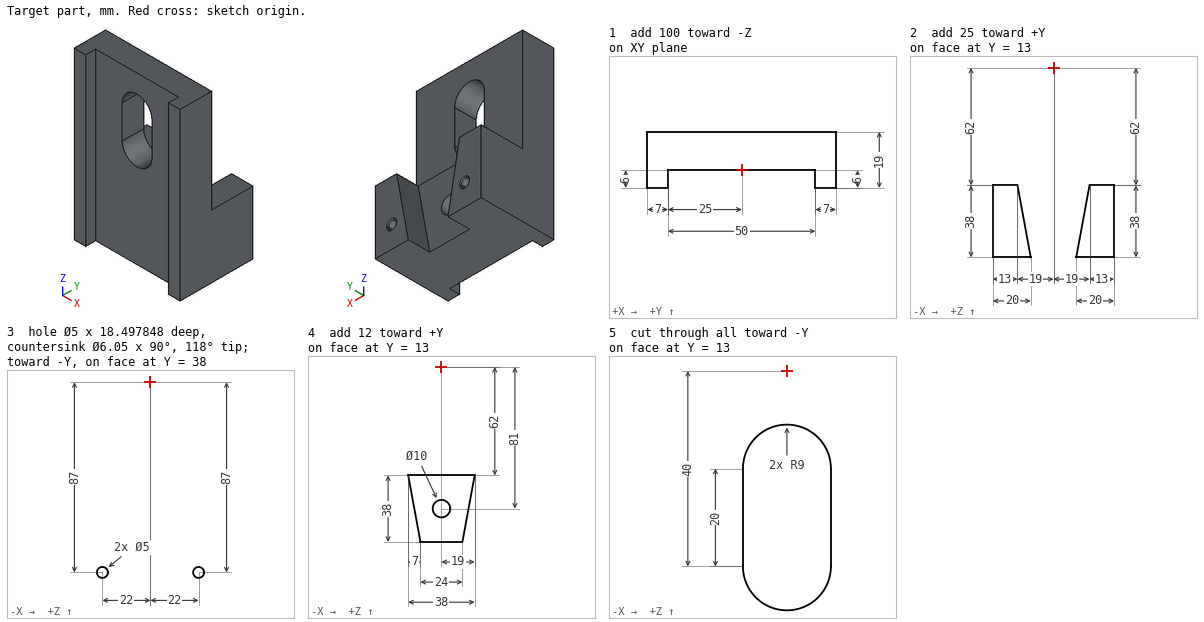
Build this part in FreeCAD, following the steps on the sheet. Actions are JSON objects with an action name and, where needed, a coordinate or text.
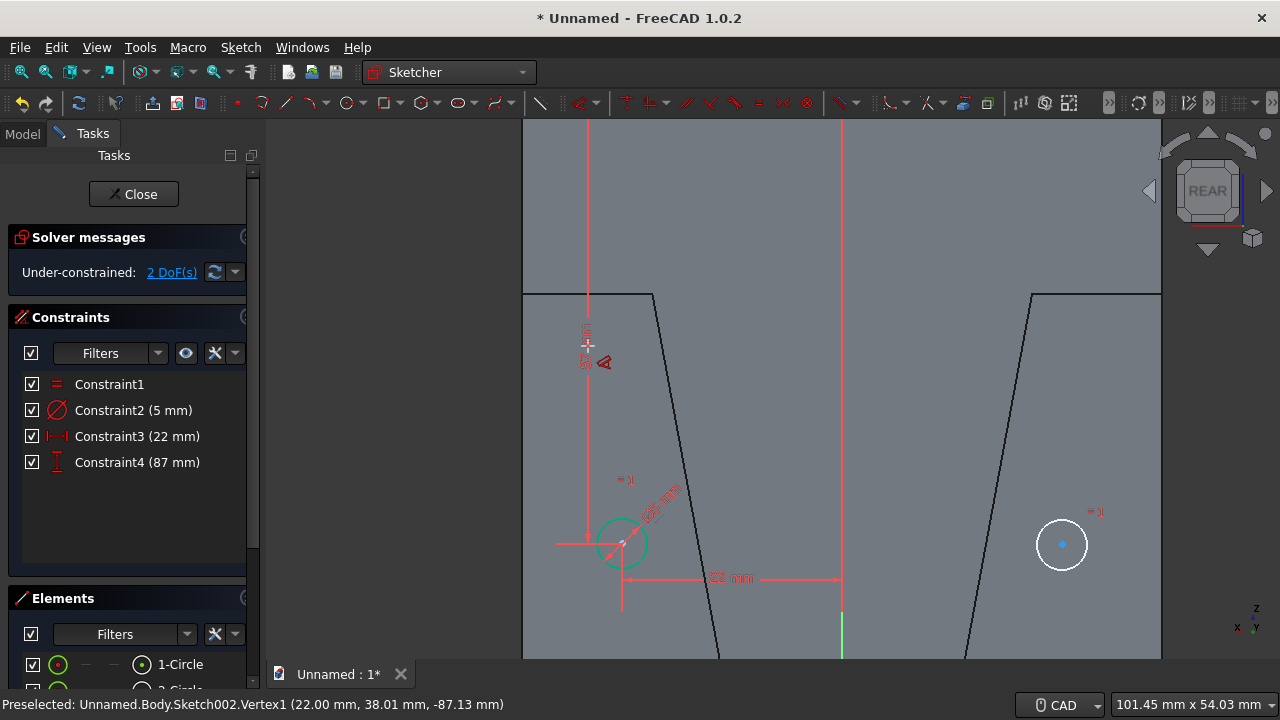
{"action": "left_click", "coordinate": [1062, 545]}
{"action": "left_click", "coordinate": [952, 579]}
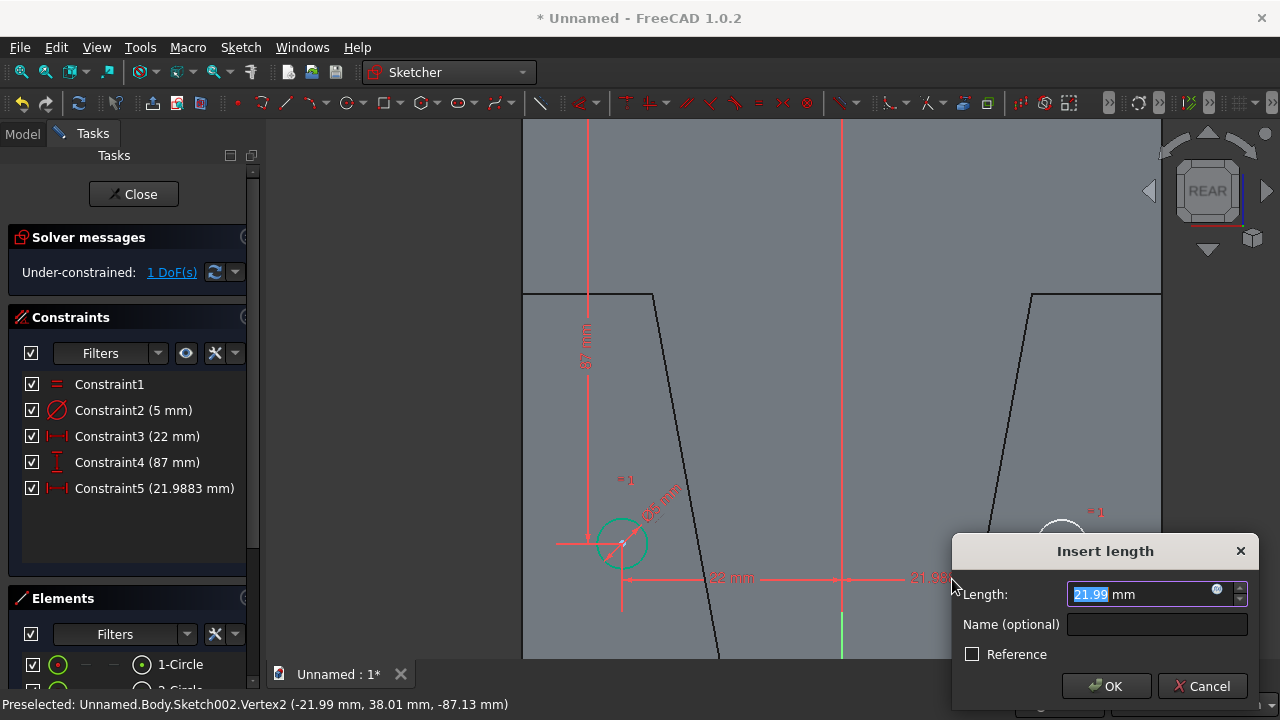
{"action": "type", "text": "22"}
{"action": "key", "text": "Return"}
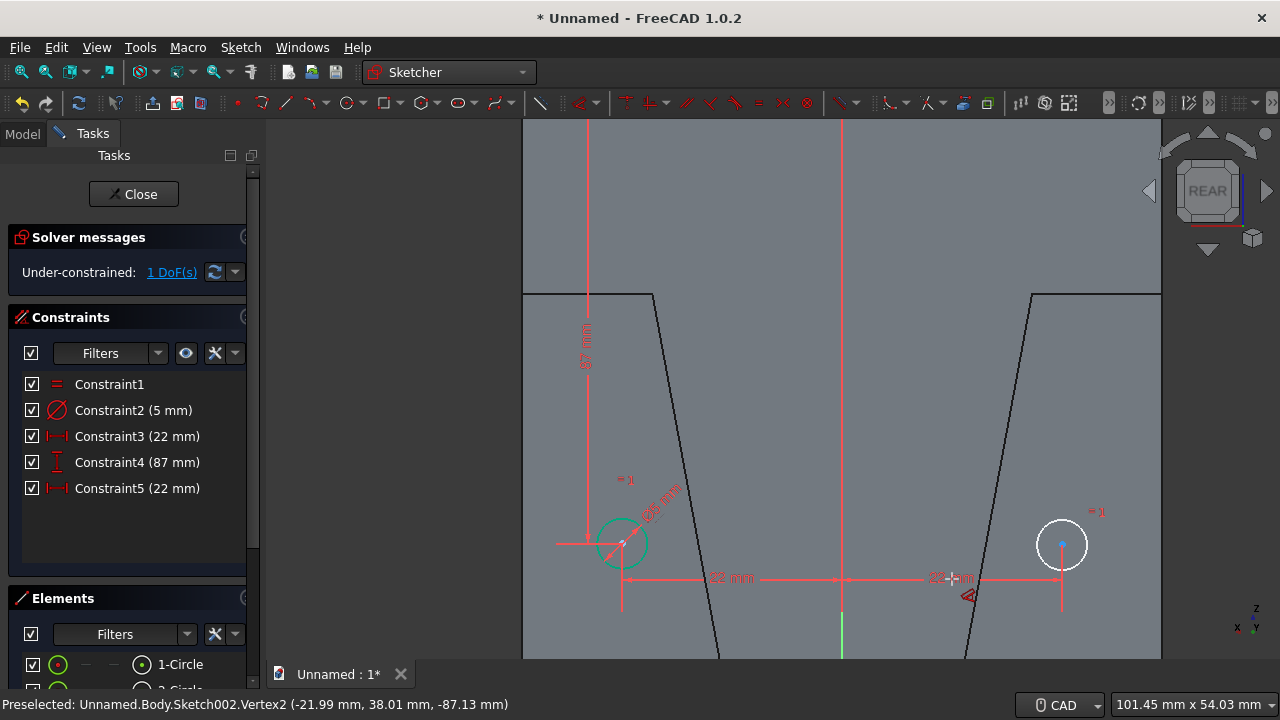
{"action": "left_click", "coordinate": [1062, 545]}
{"action": "left_click", "coordinate": [1096, 346]}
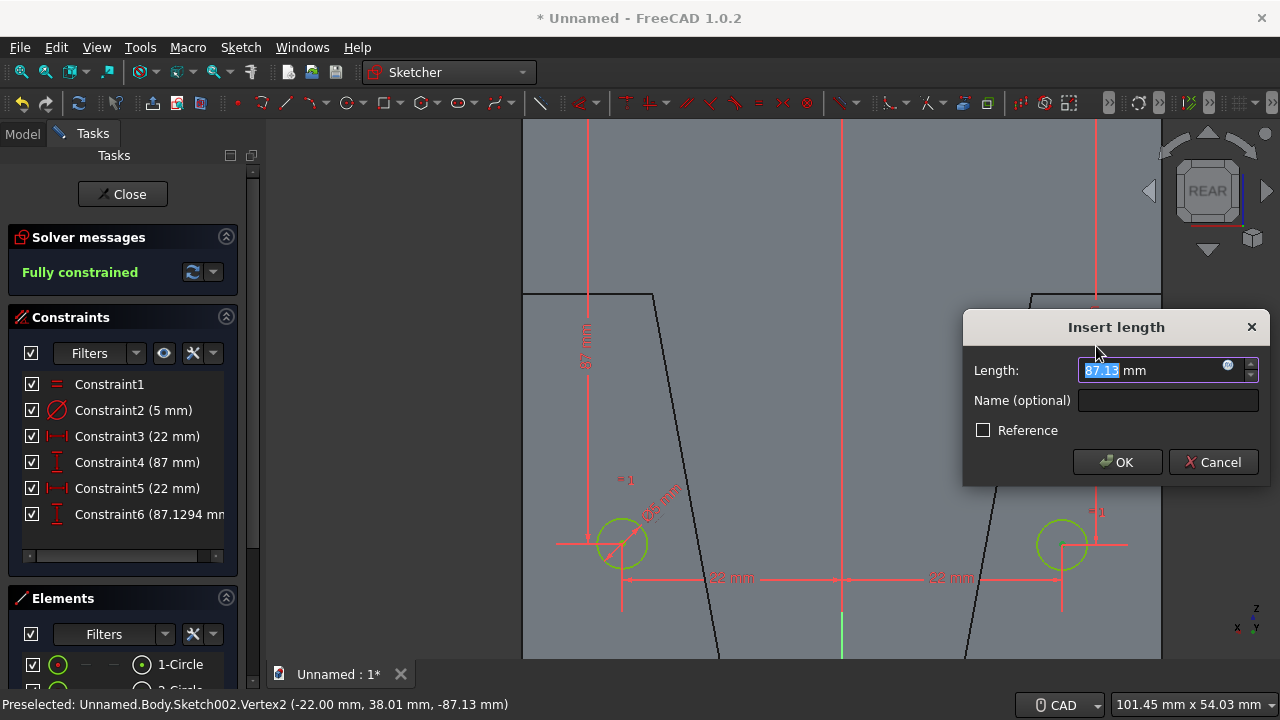
{"action": "type", "text": "87"}
{"action": "key", "text": "Return"}
{"action": "key", "text": "Escape"}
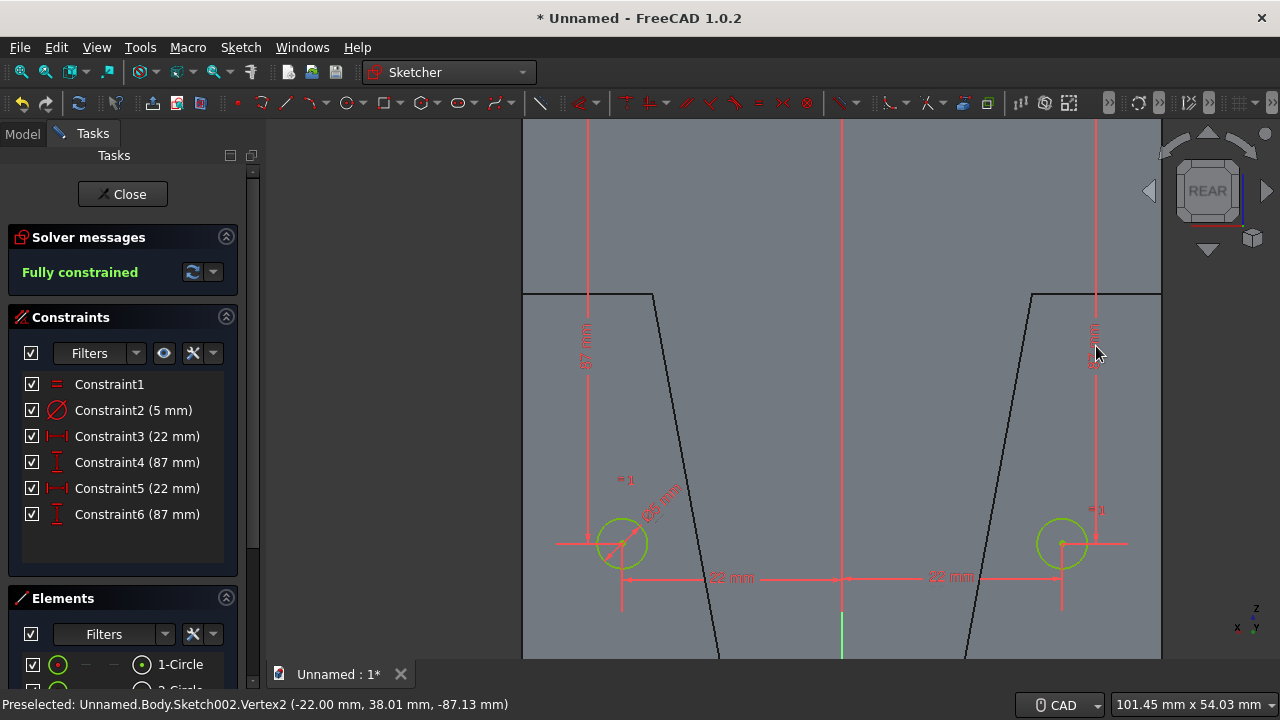
{"action": "left_click", "coordinate": [123, 194]}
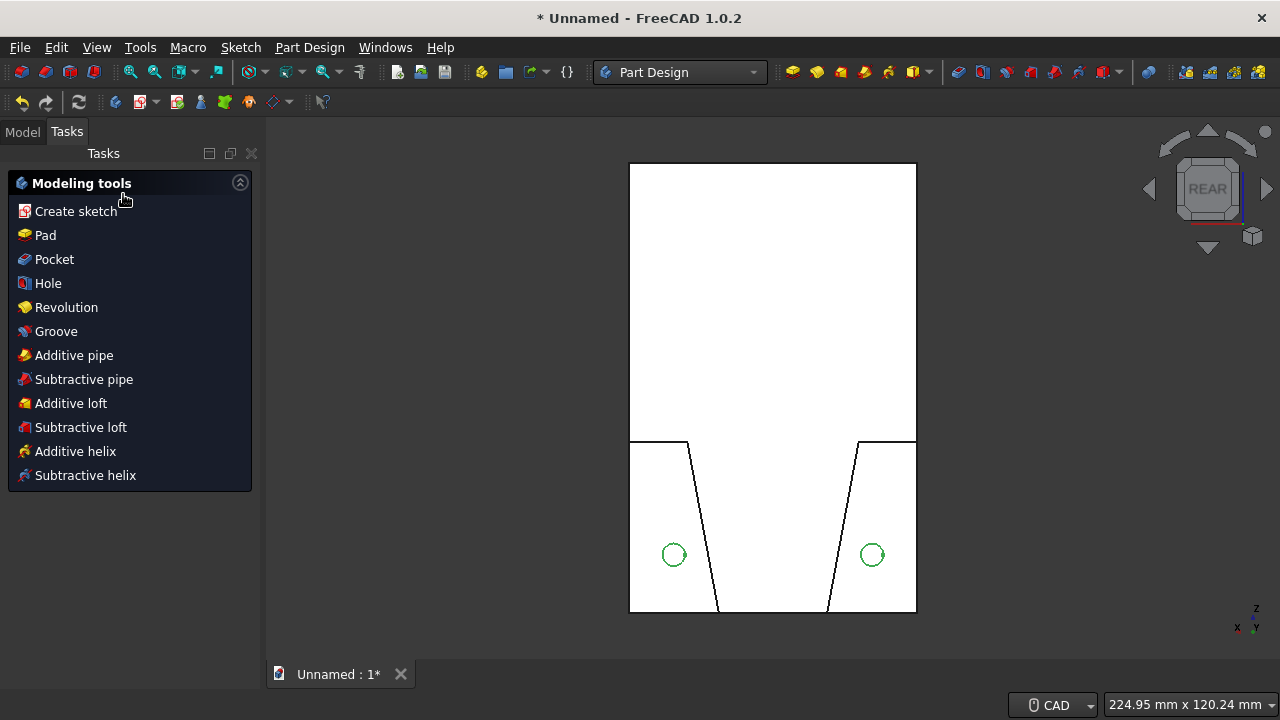
{"action": "left_click", "coordinate": [984, 72]}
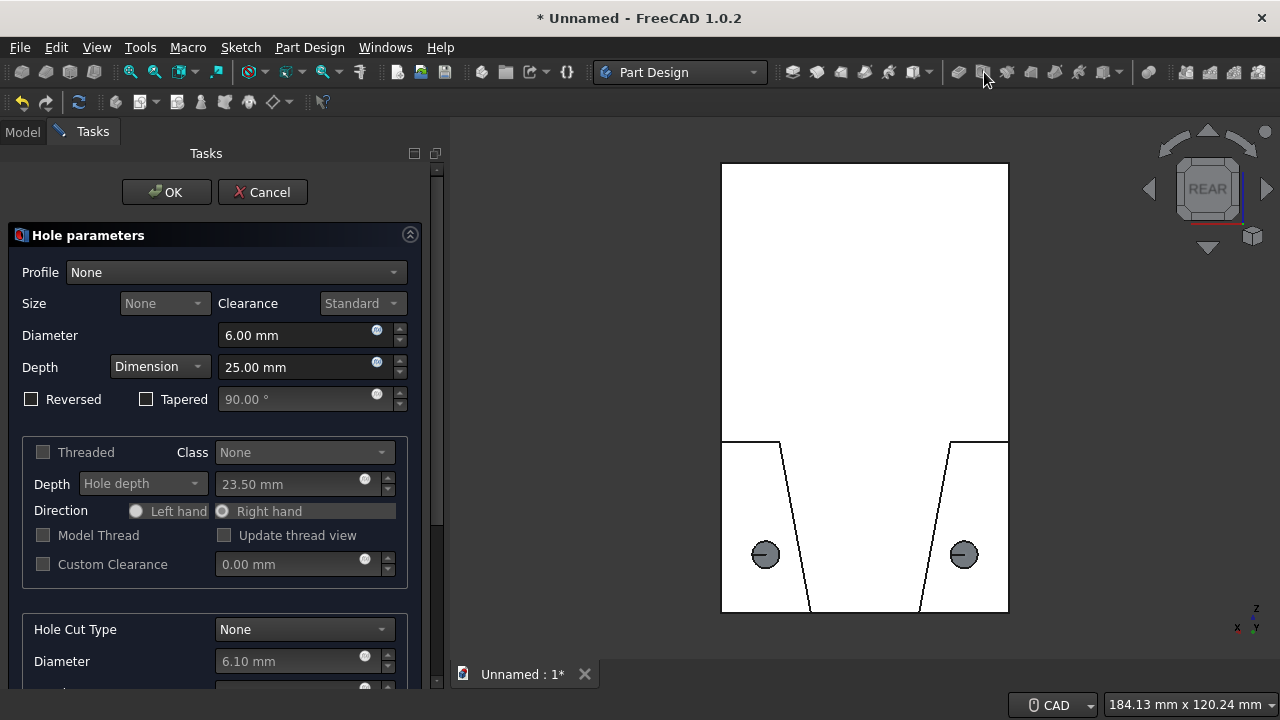
{"action": "triple_click", "coordinate": [305, 335]}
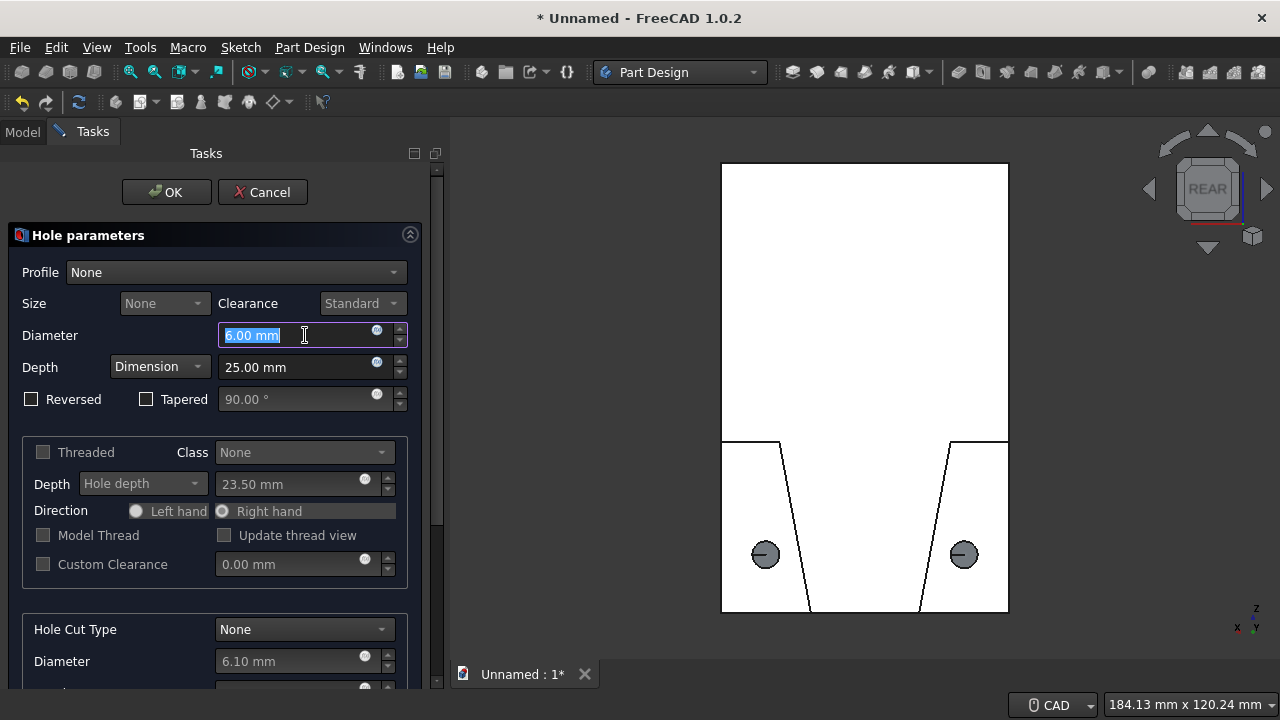
{"action": "type", "text": "5"}
{"action": "key", "text": "Tab"}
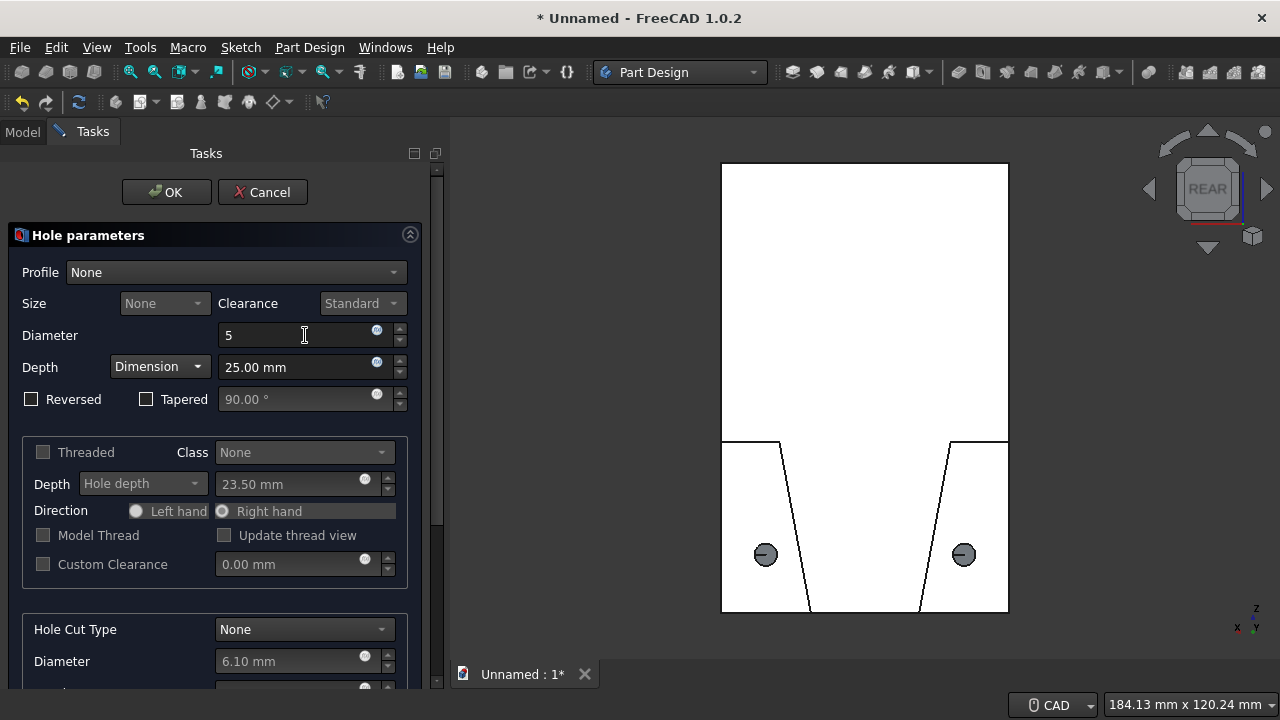
{"action": "triple_click", "coordinate": [305, 367]}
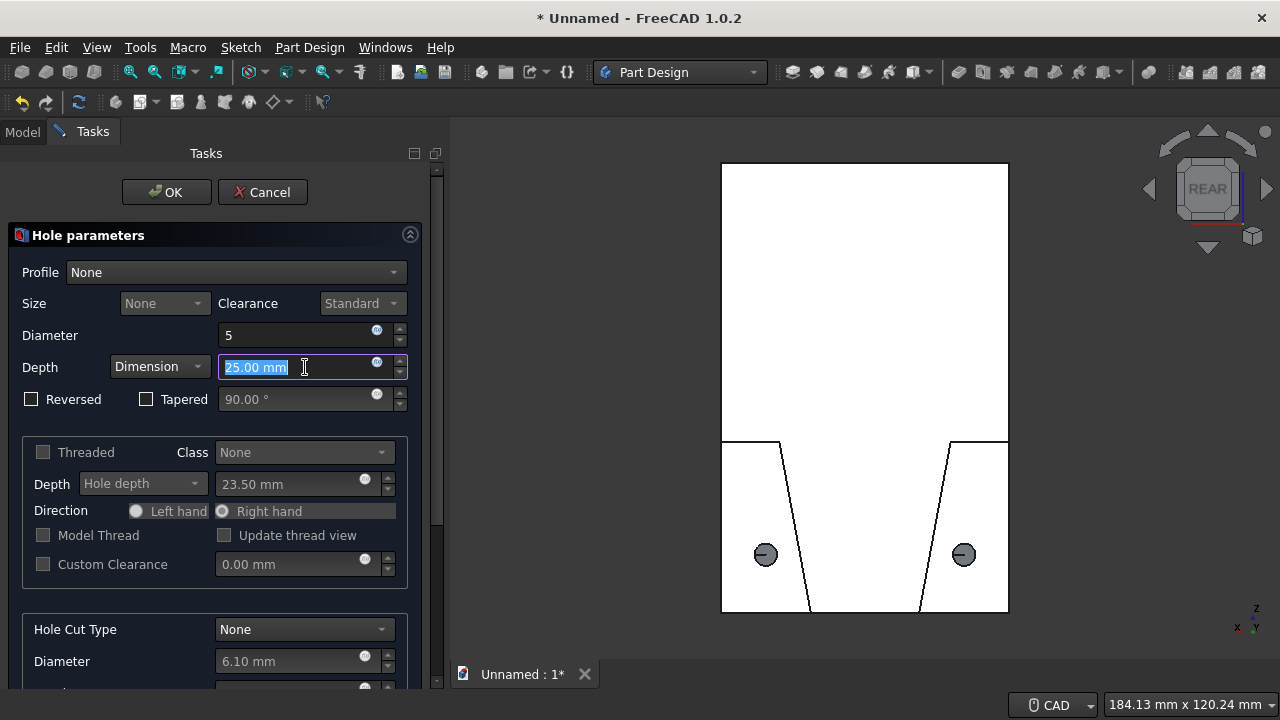
{"action": "type", "text": "18.497848"}
{"action": "key", "text": "Tab"}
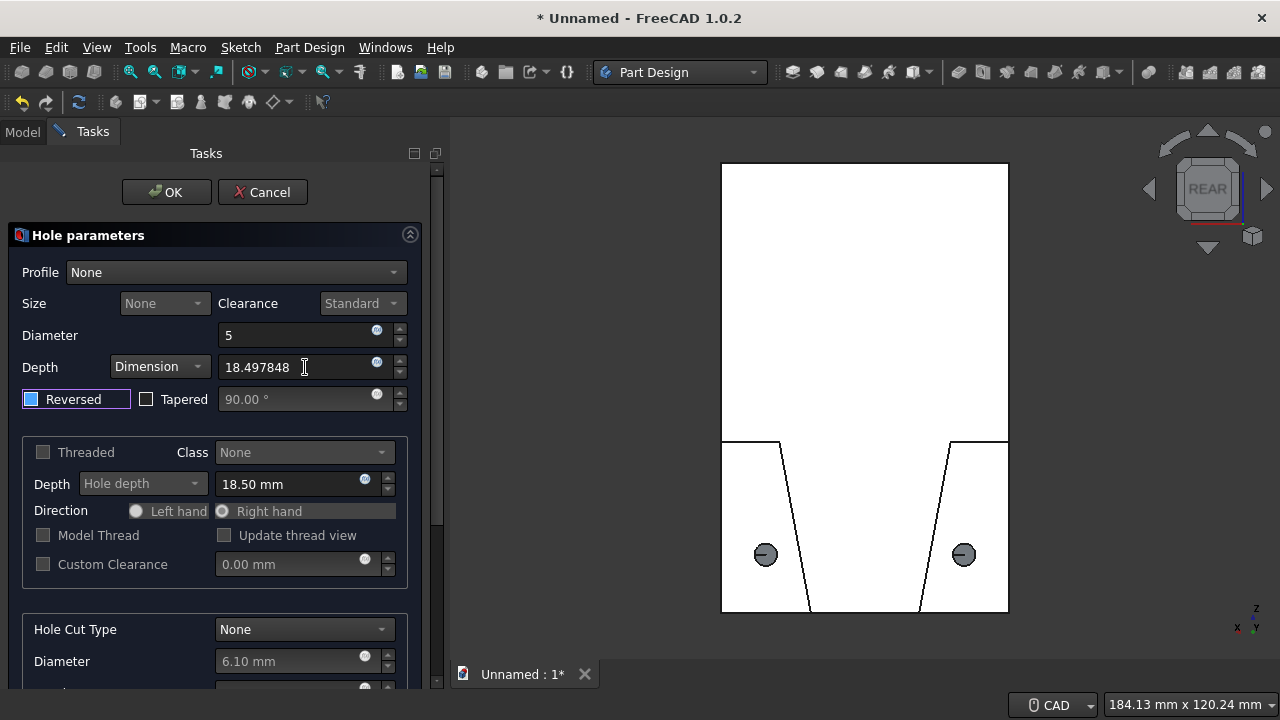
{"action": "left_click", "coordinate": [306, 630]}